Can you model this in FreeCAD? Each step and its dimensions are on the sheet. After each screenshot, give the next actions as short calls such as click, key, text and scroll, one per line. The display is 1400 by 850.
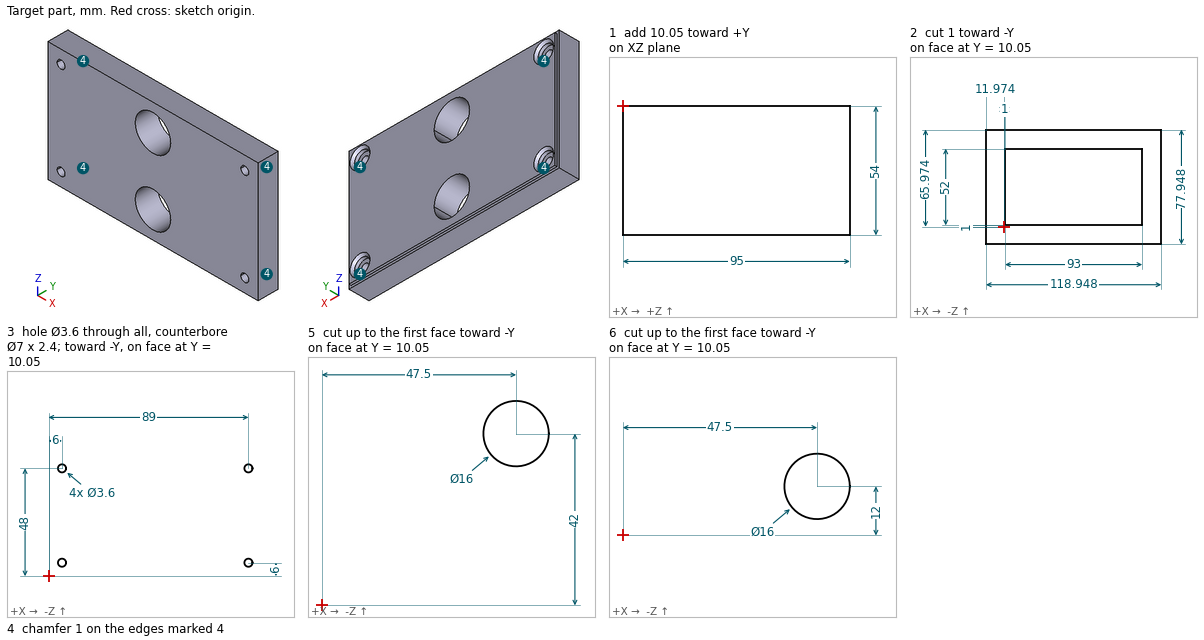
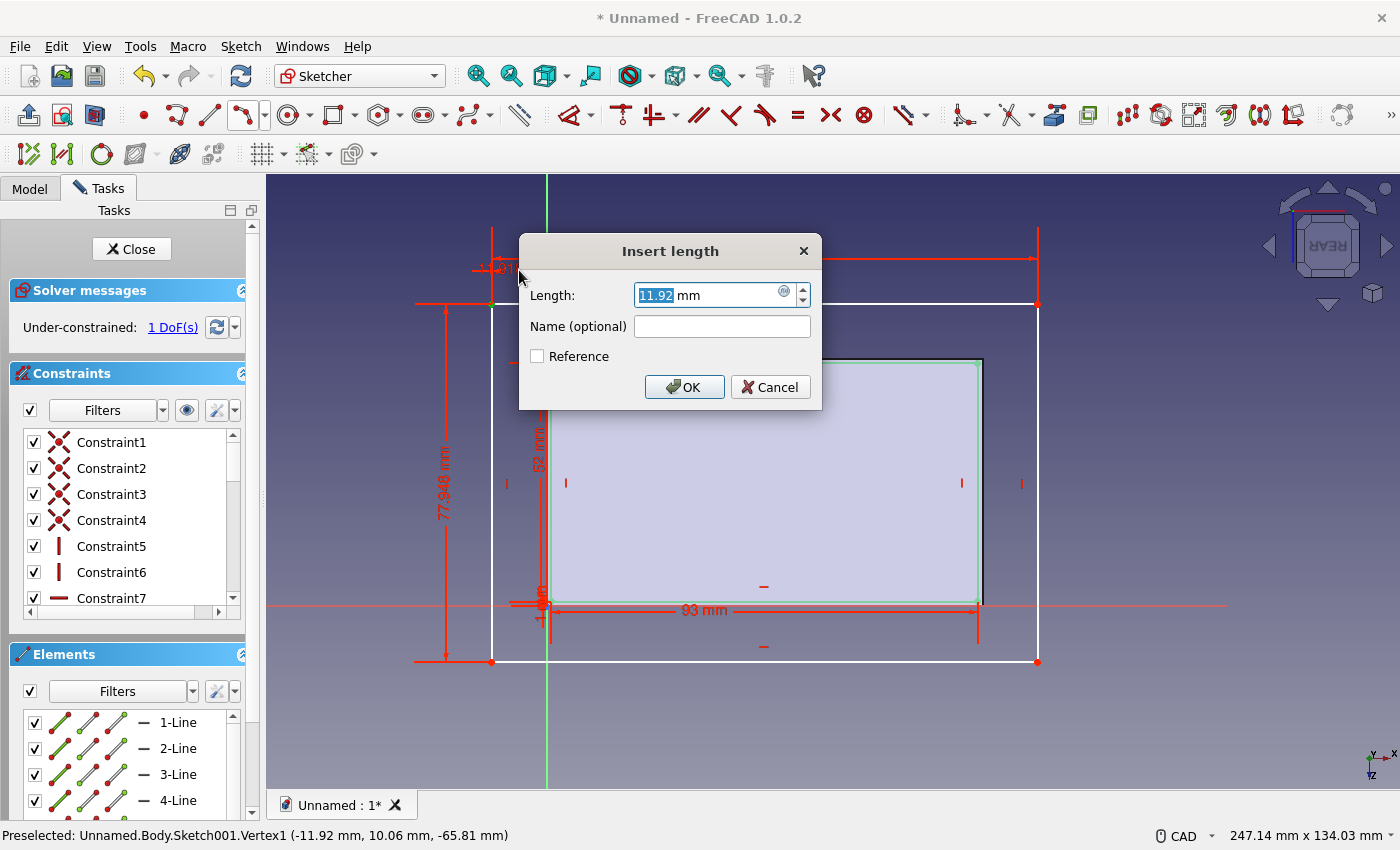
text(11.974)
key(Return)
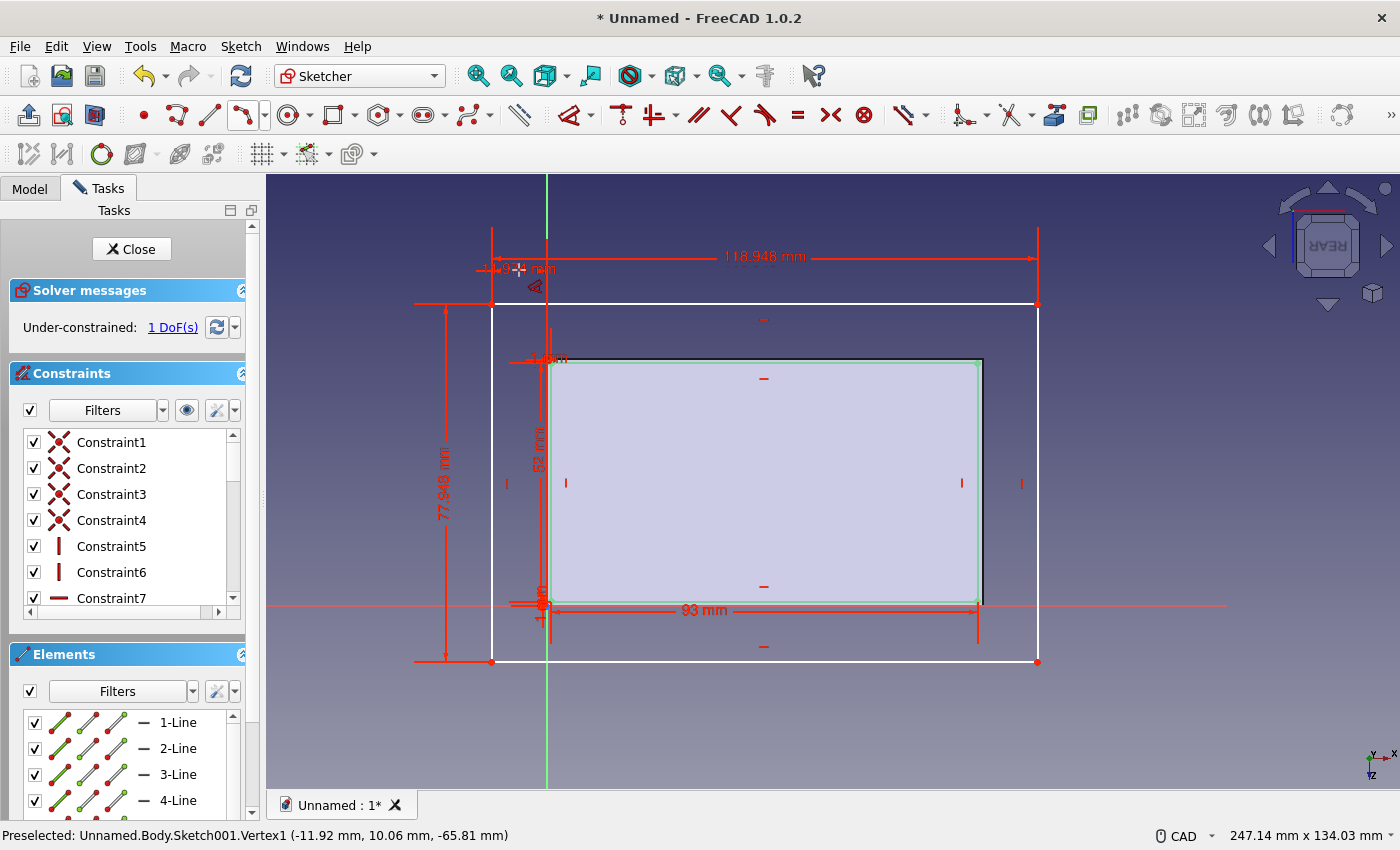
click(492, 304)
click(458, 455)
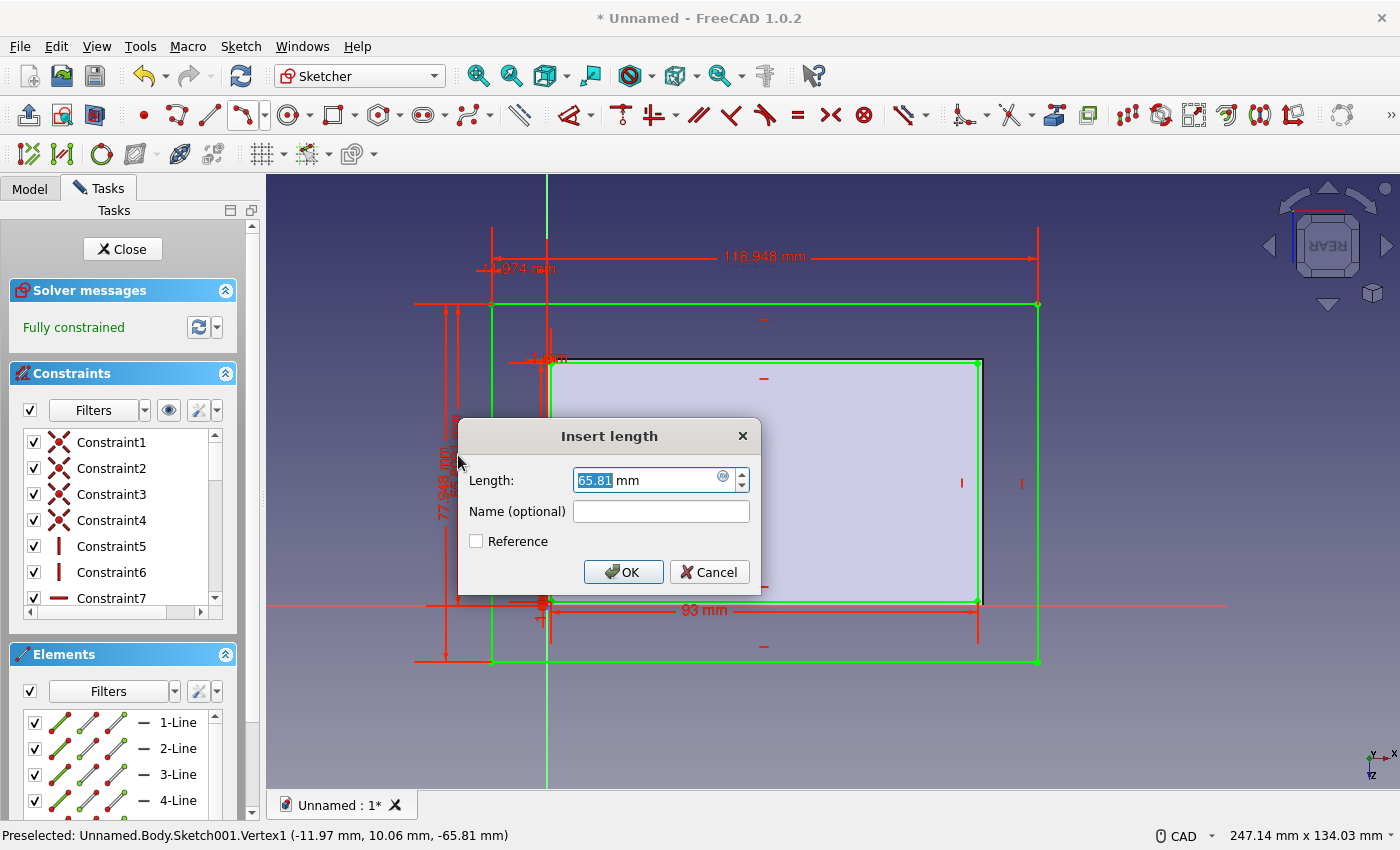
text(65.974)
key(Return)
key(Escape)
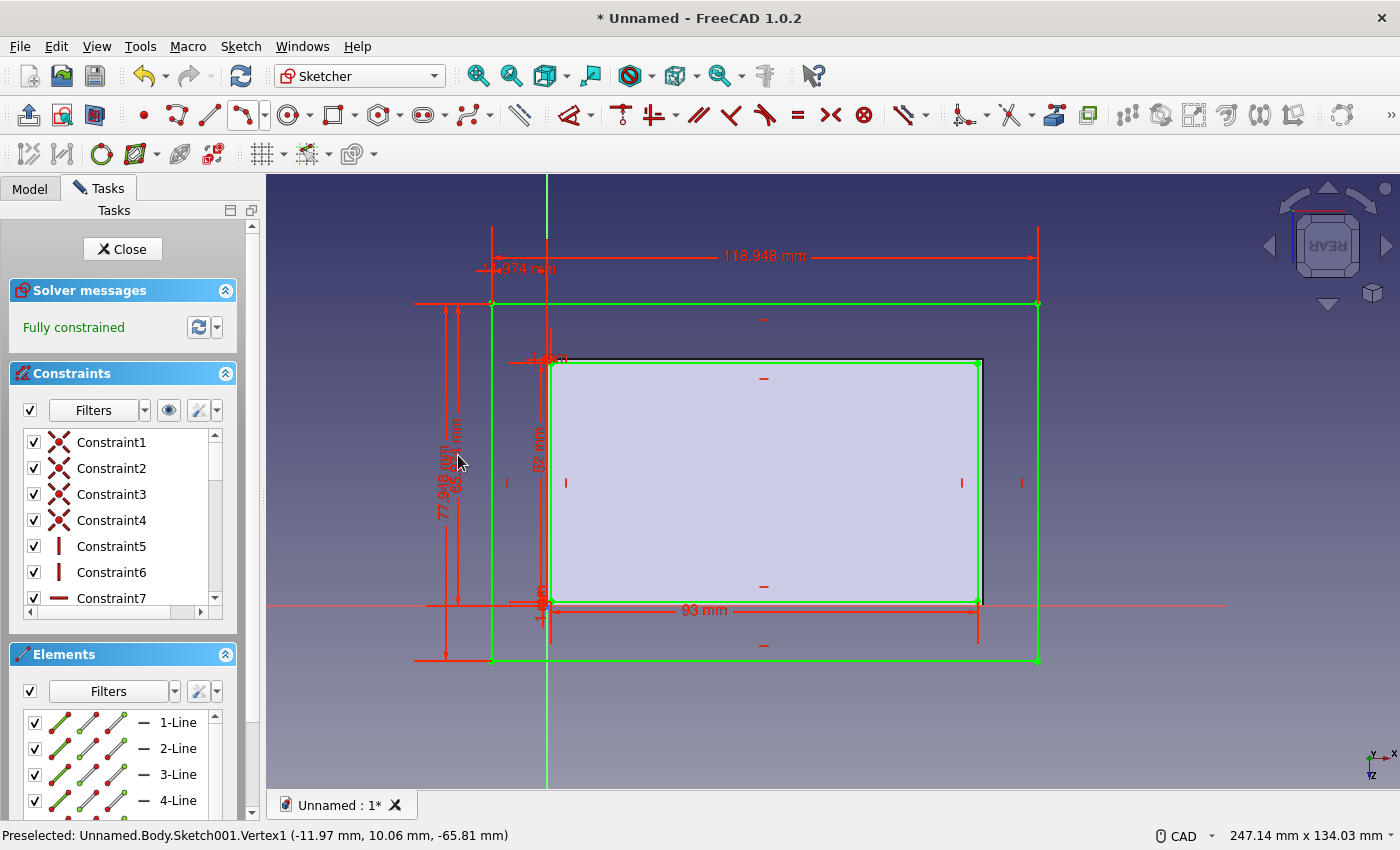
click(123, 249)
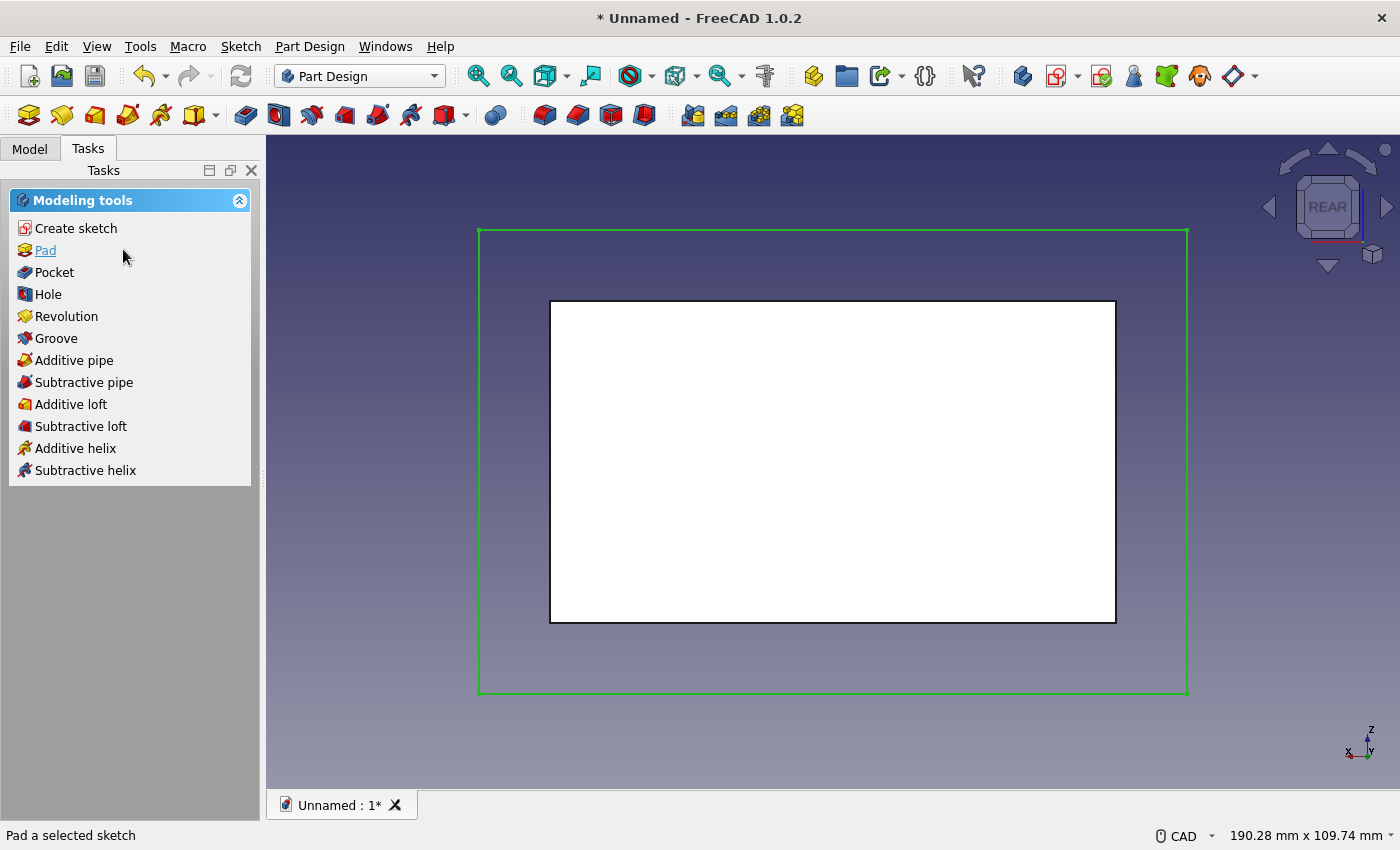
click(246, 116)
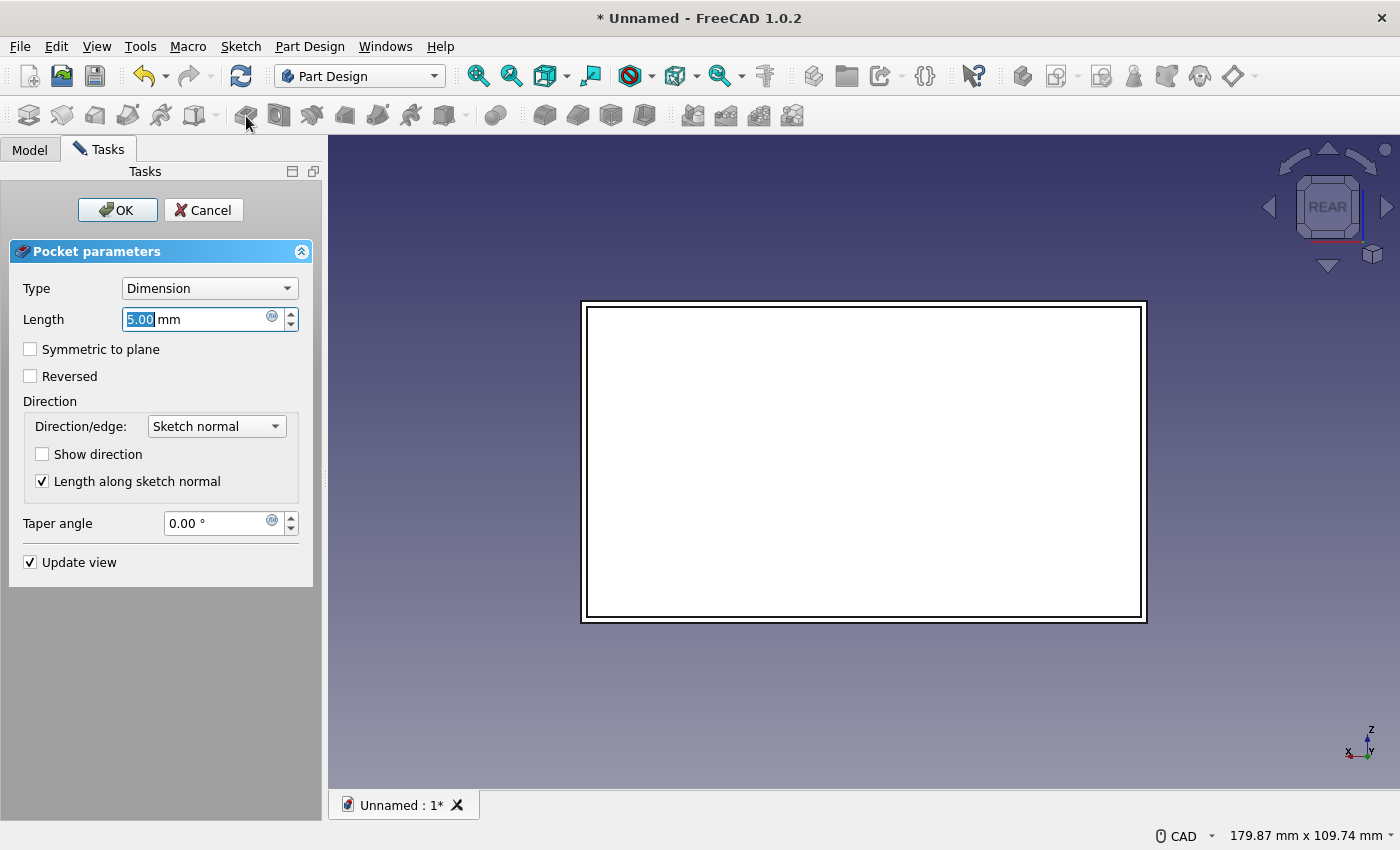
text(1)
key(Tab)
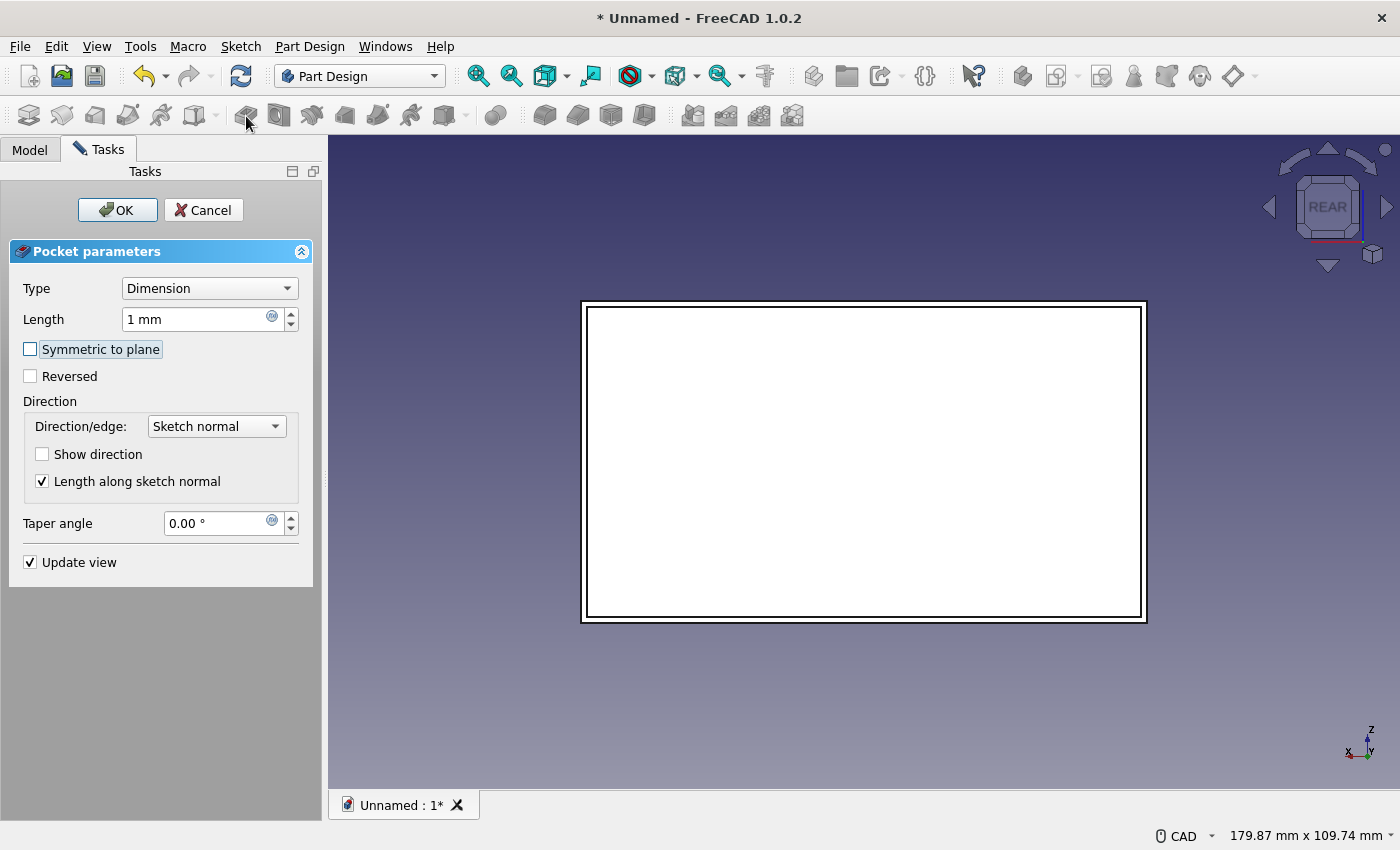
click(118, 210)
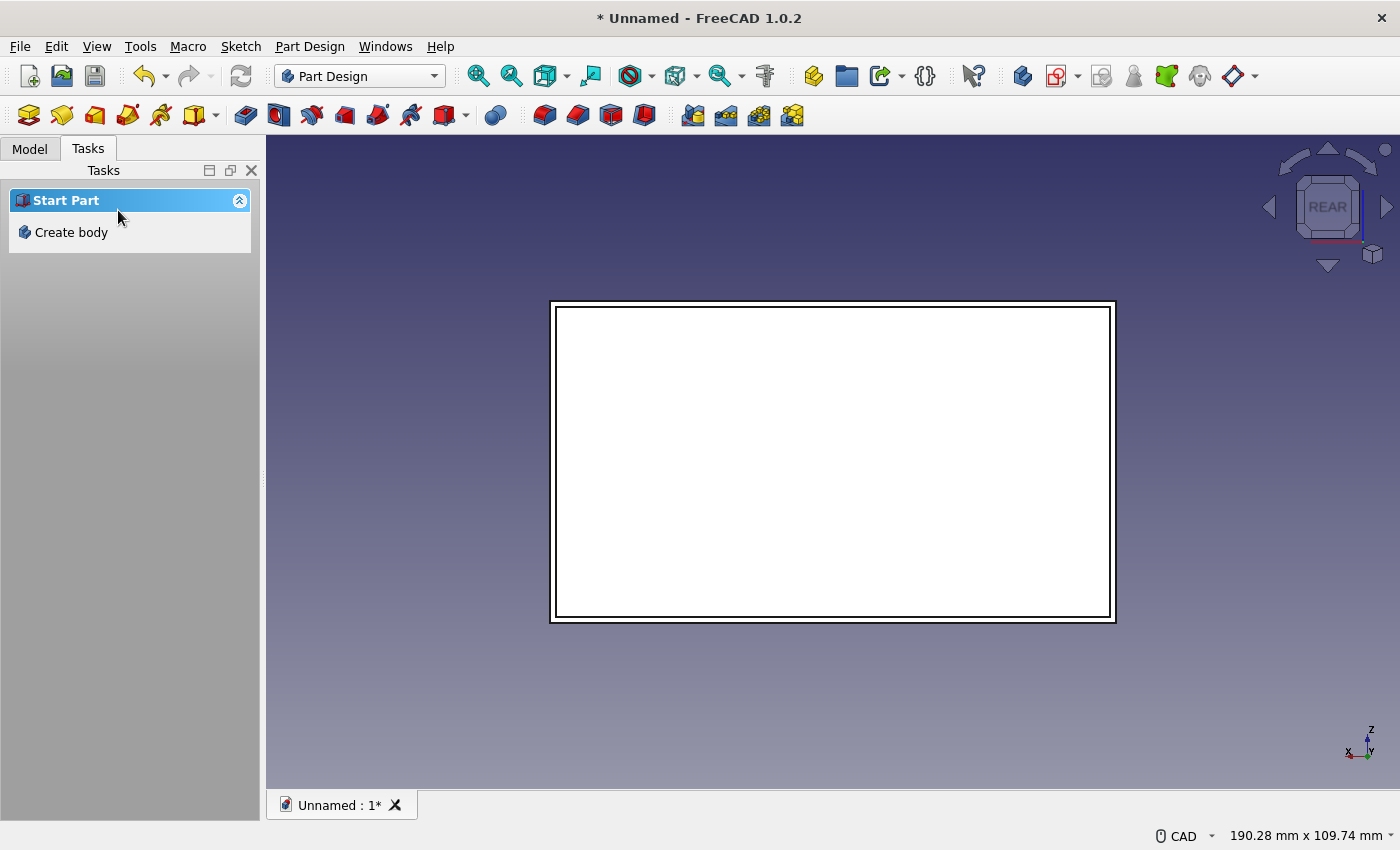
click(754, 461)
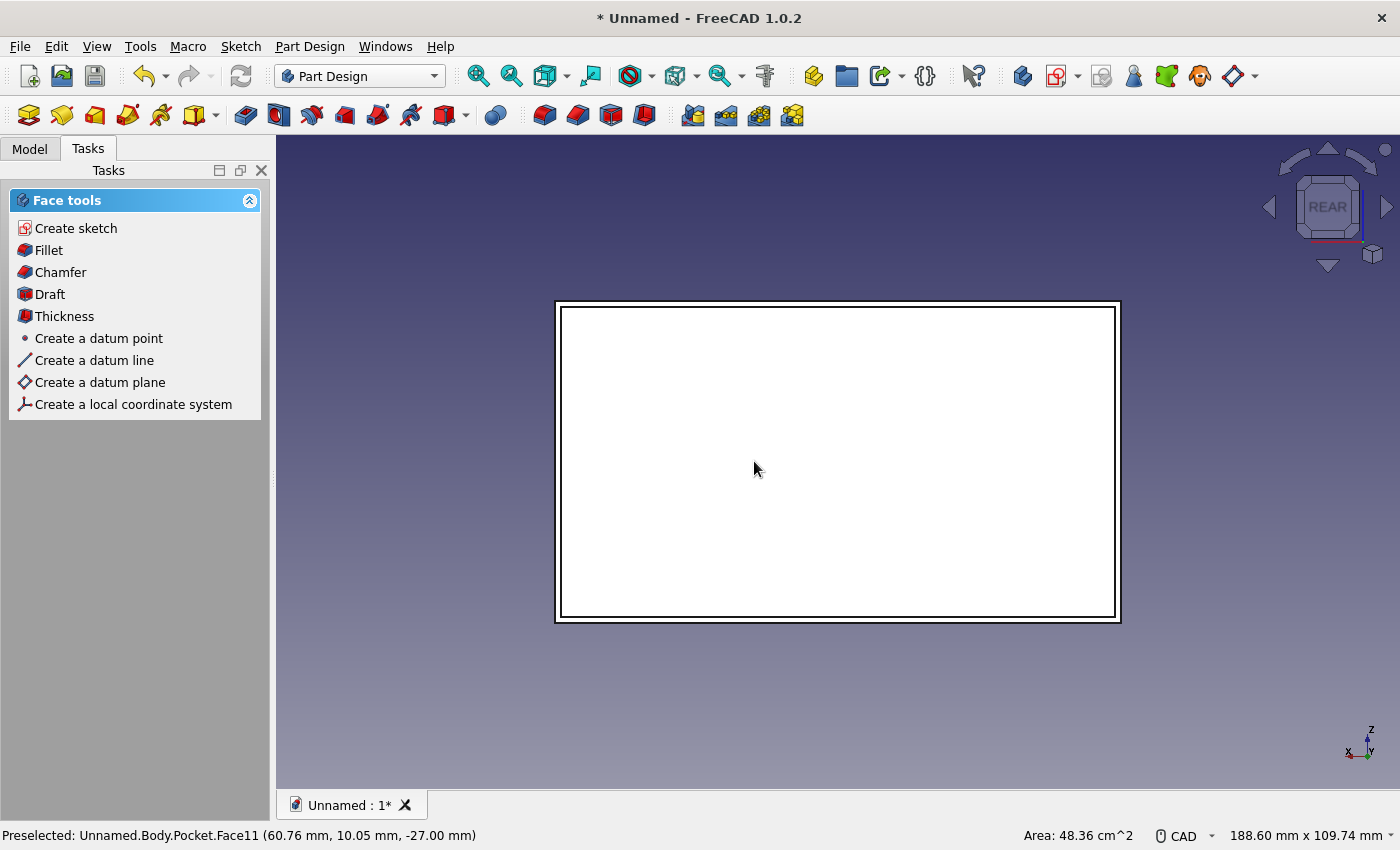
click(1056, 76)